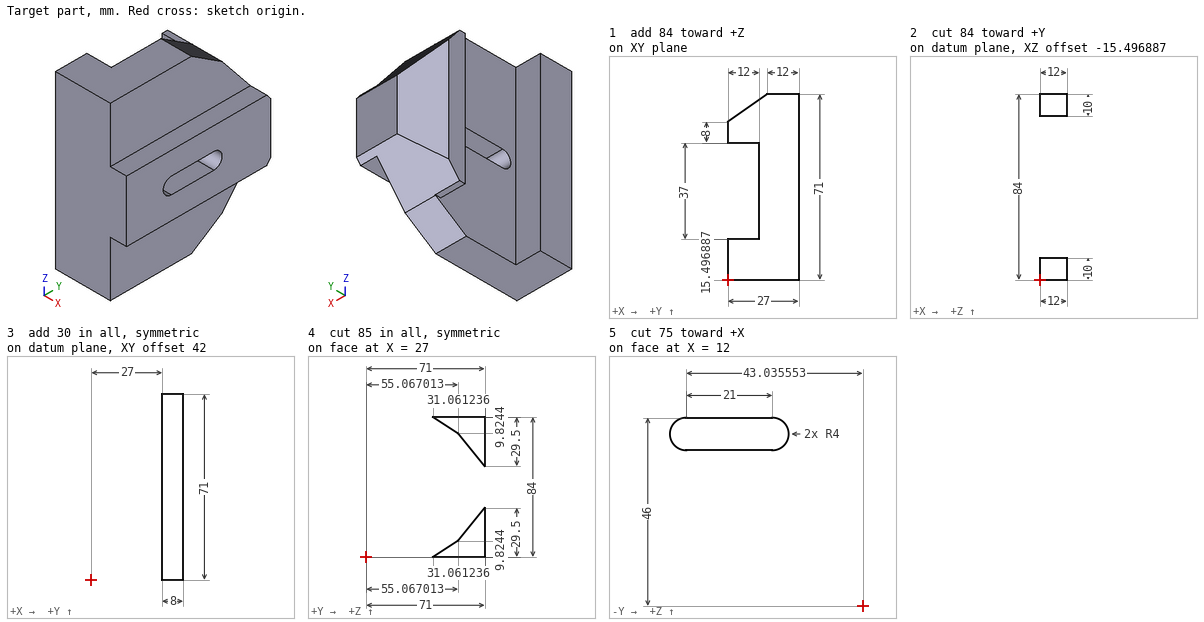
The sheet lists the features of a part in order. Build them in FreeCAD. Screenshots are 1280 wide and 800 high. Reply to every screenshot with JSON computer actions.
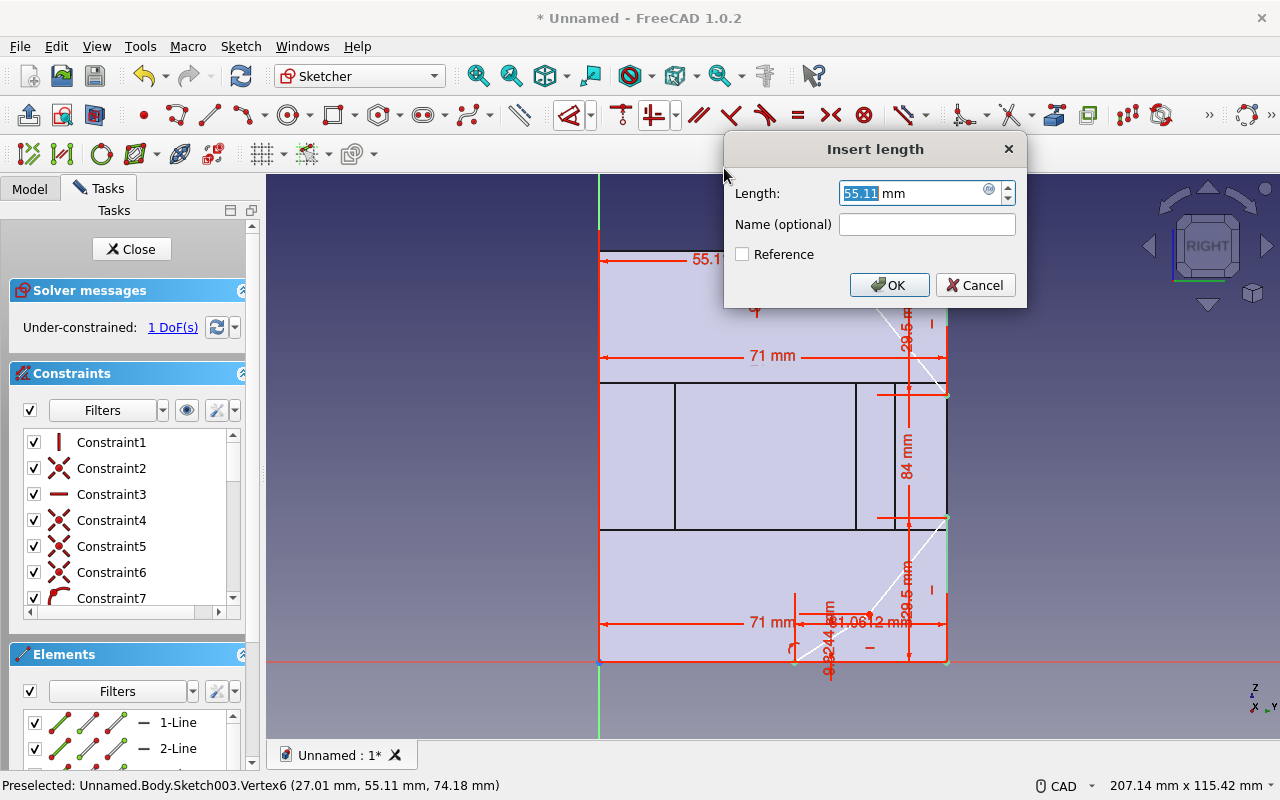
{"action": "type", "text": "55.067013"}
{"action": "key", "text": "Return"}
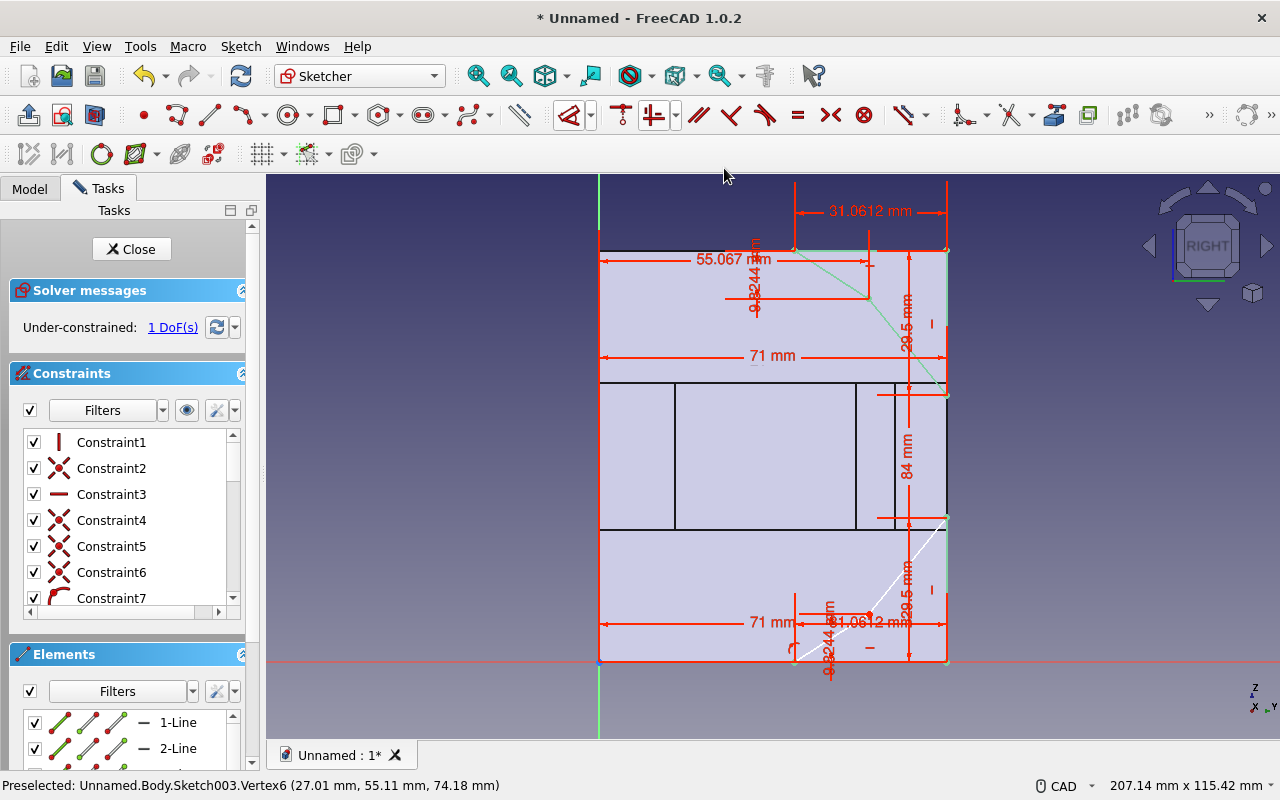
{"action": "left_click", "coordinate": [869, 614]}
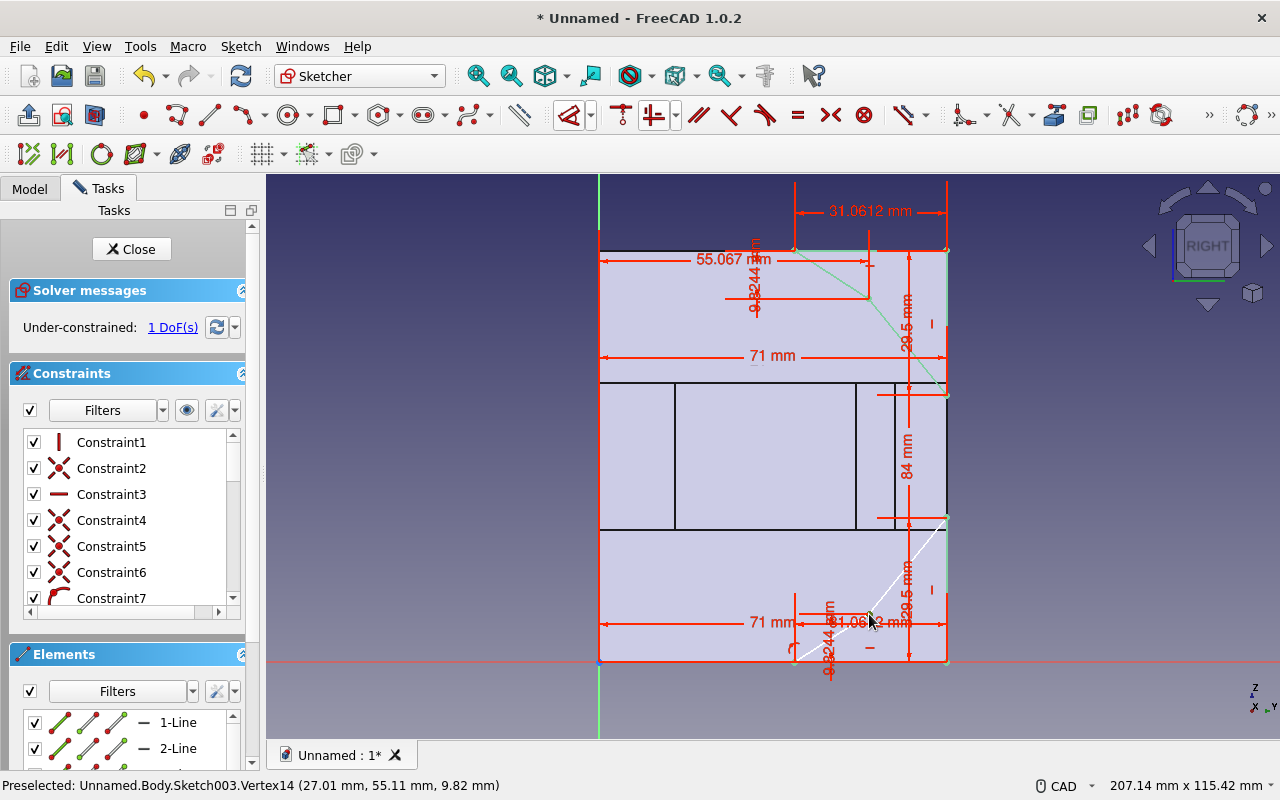
{"action": "key", "text": "l"}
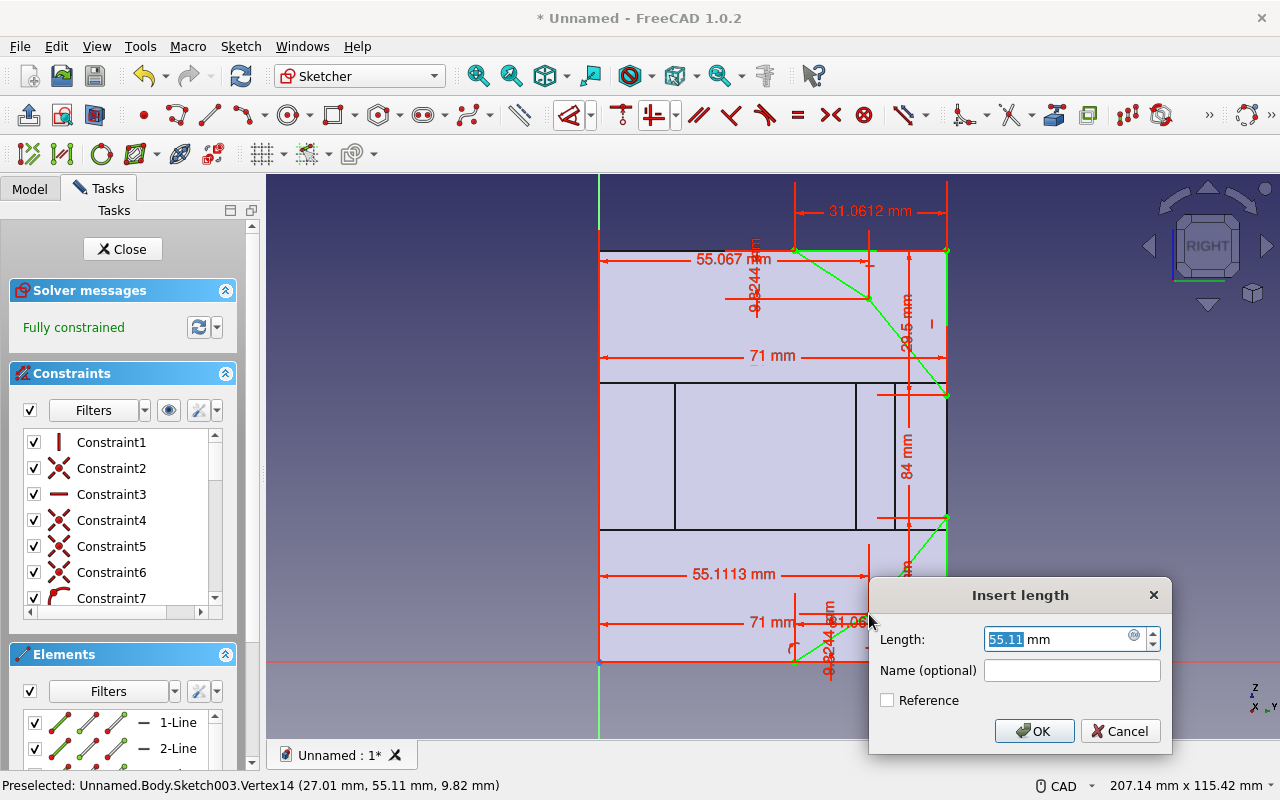
{"action": "type", "text": "55.067013"}
{"action": "key", "text": "Return"}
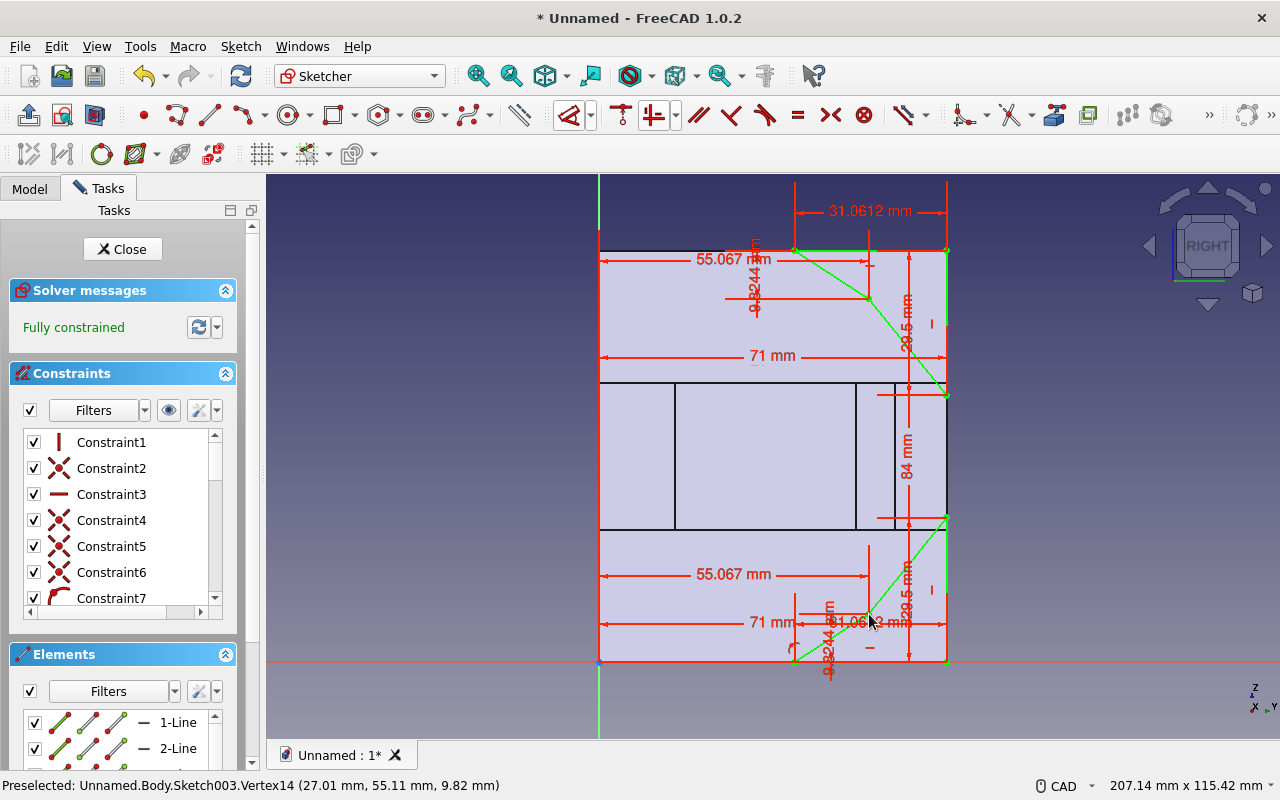
{"action": "left_click", "coordinate": [123, 249]}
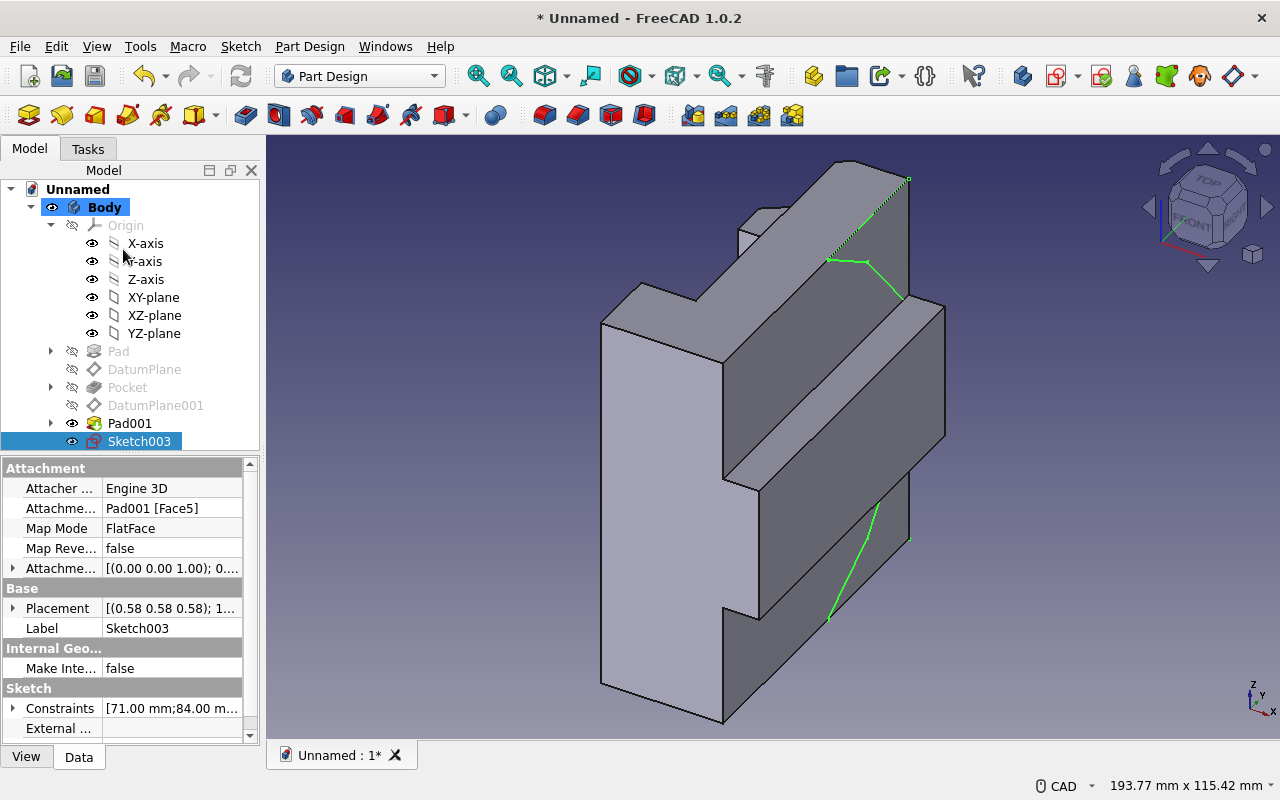
{"action": "left_click", "coordinate": [246, 116]}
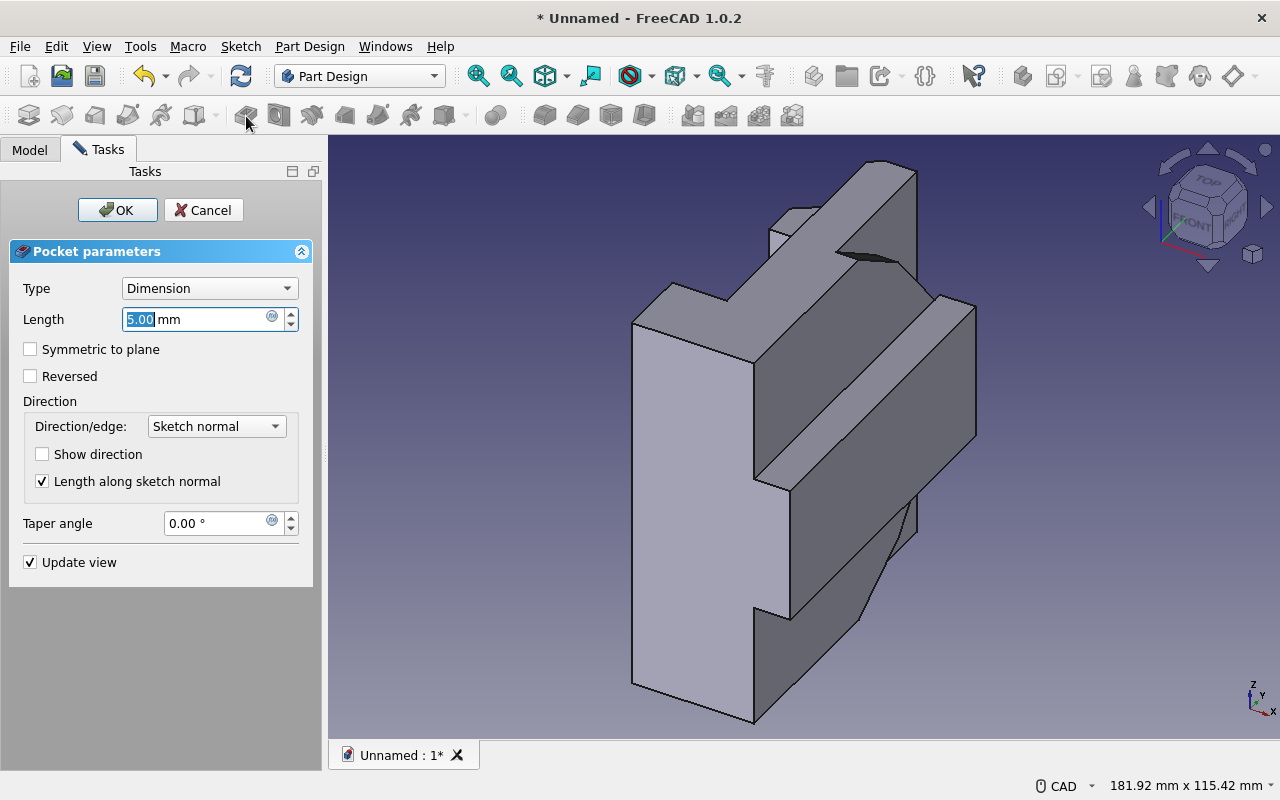
{"action": "type", "text": "85"}
{"action": "key", "text": "Tab"}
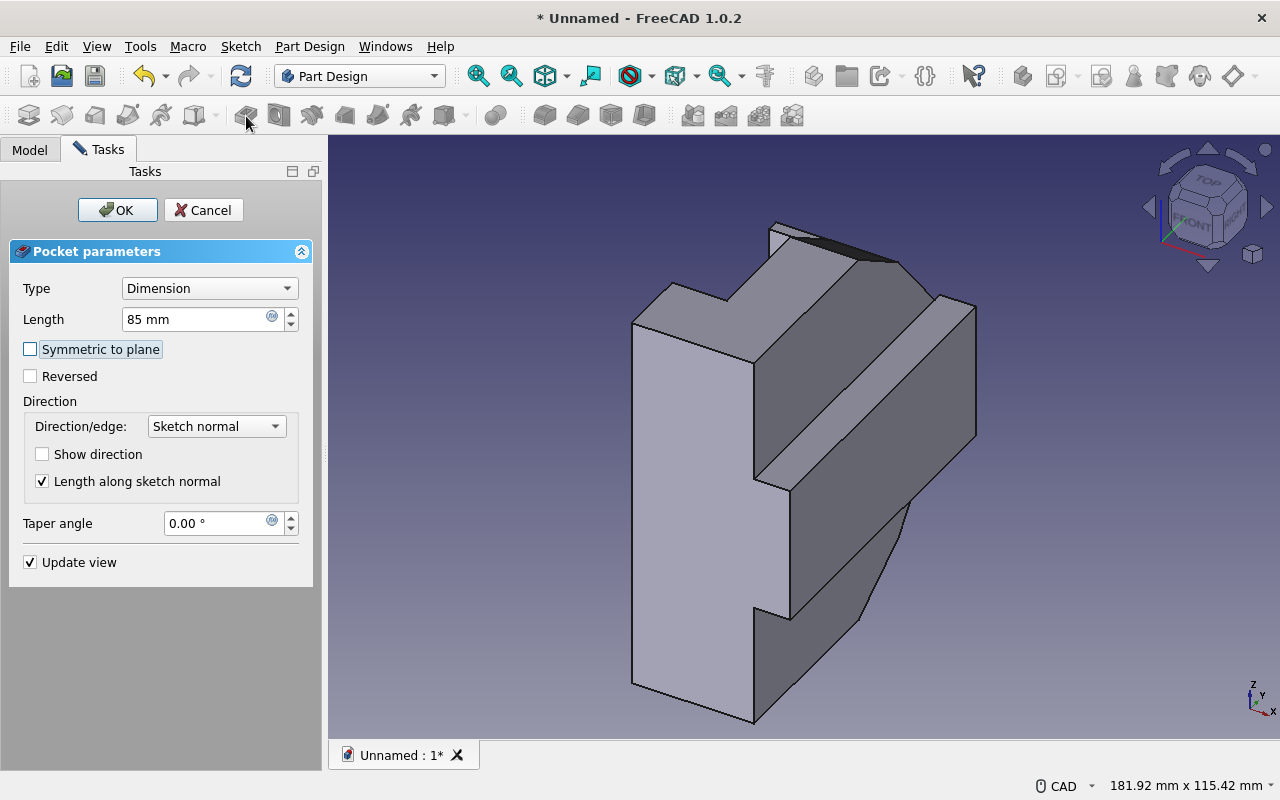
{"action": "left_click", "coordinate": [31, 349]}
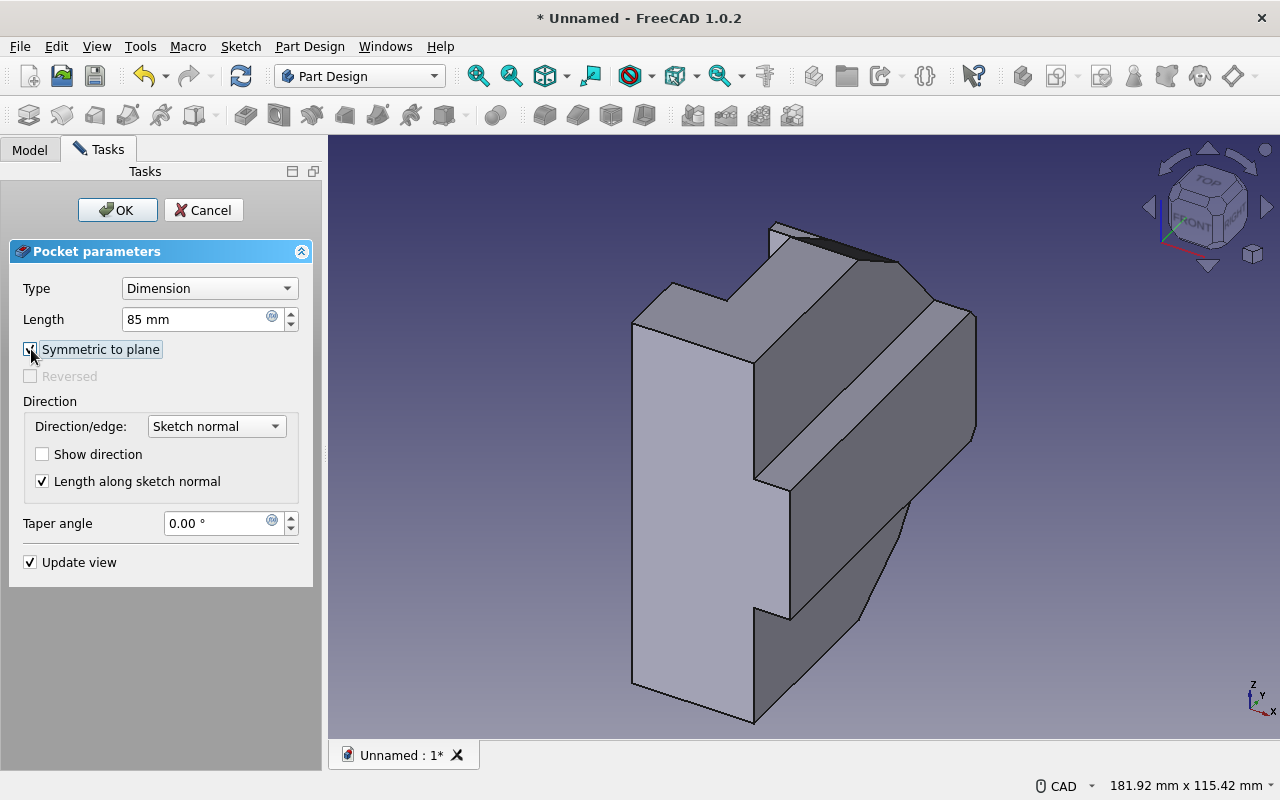
{"action": "left_click", "coordinate": [118, 210]}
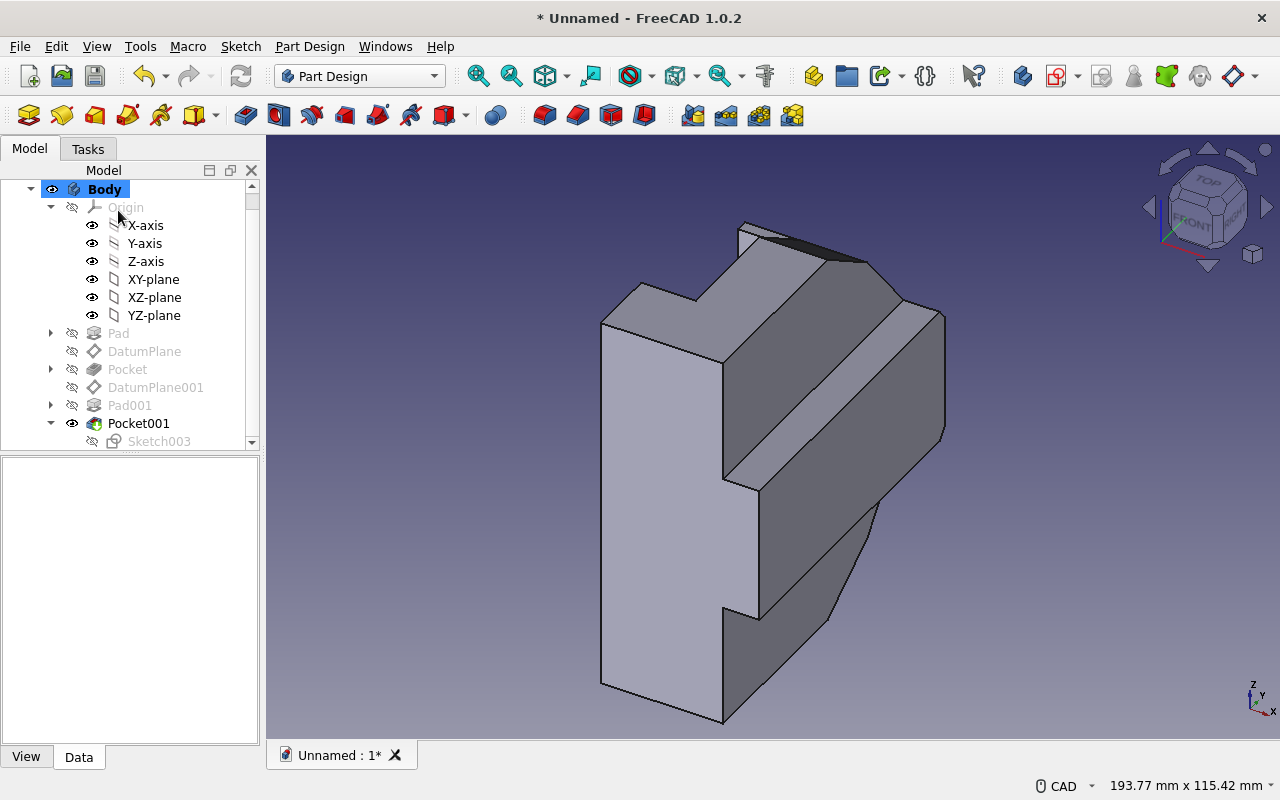
{"action": "key", "text": "6"}